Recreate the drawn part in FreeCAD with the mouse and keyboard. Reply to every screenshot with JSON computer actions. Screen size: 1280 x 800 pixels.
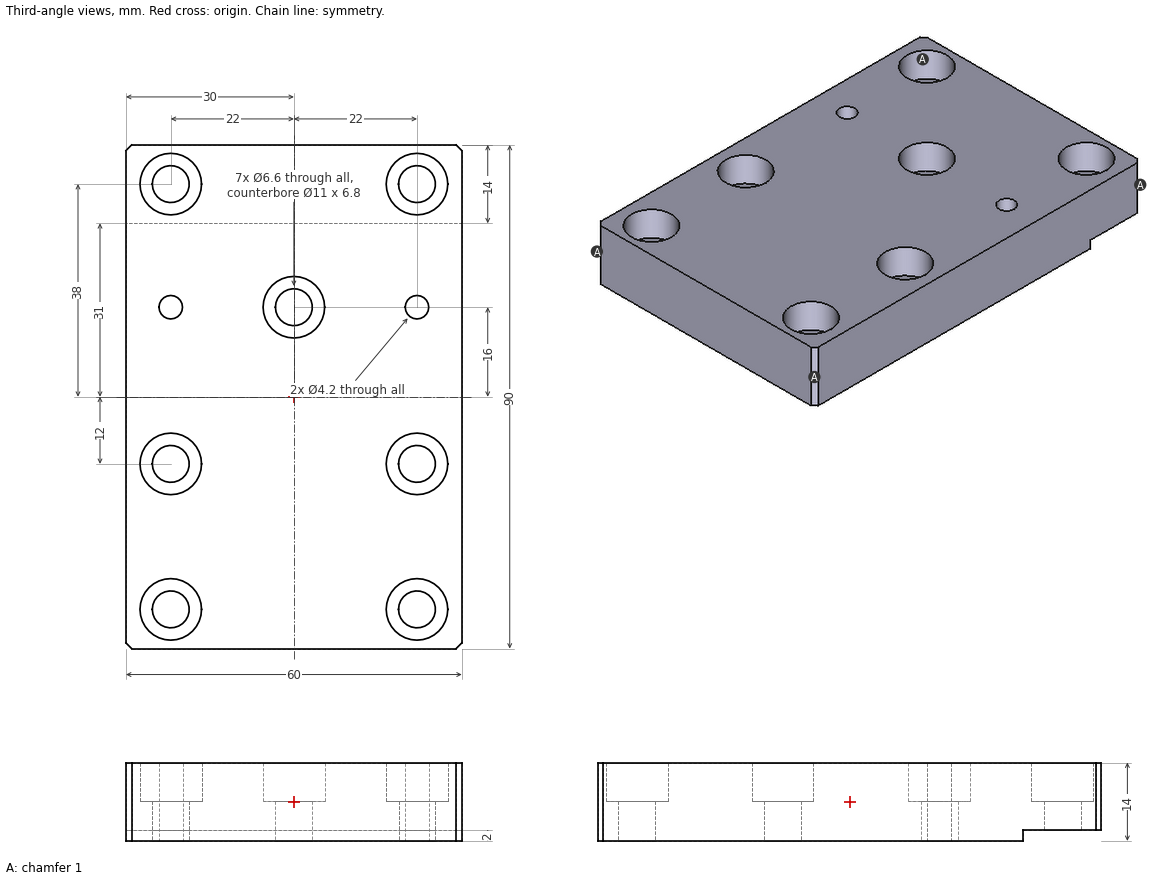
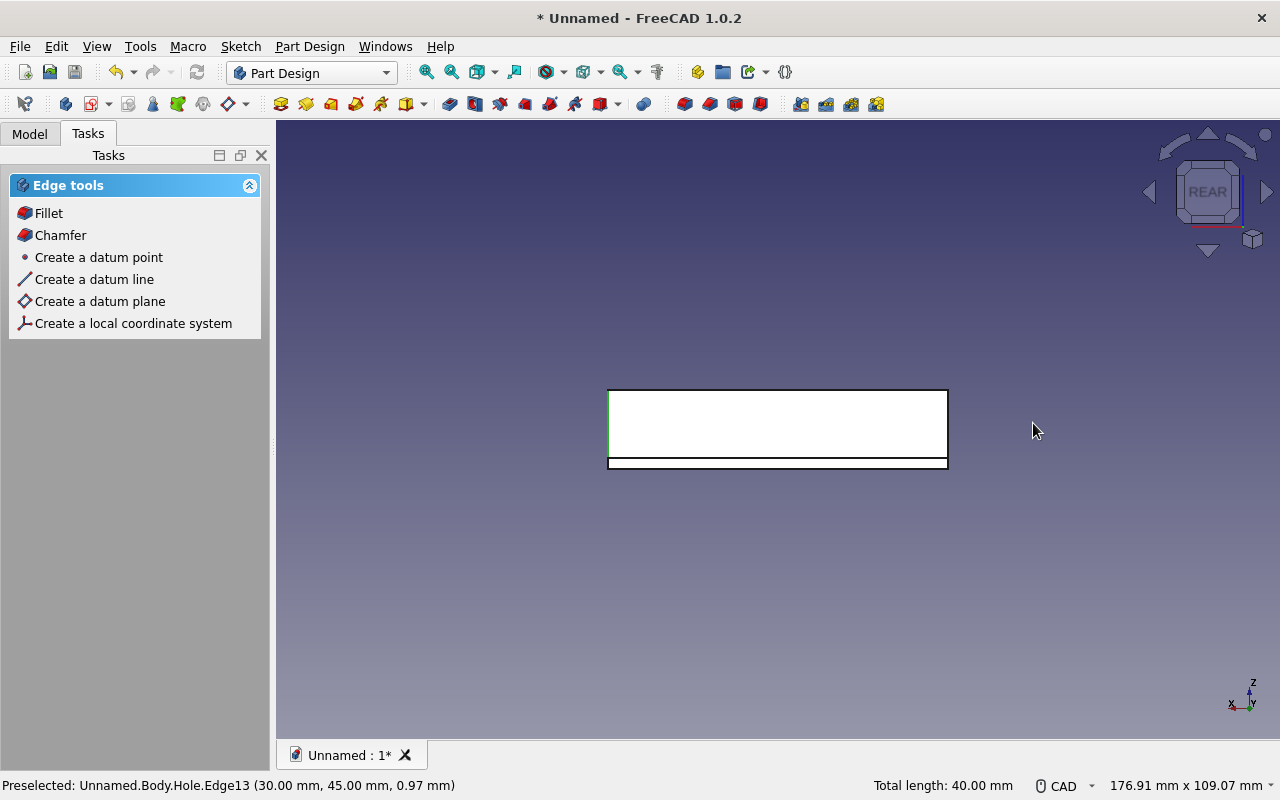
{"action": "left_click", "coordinate": [427, 72]}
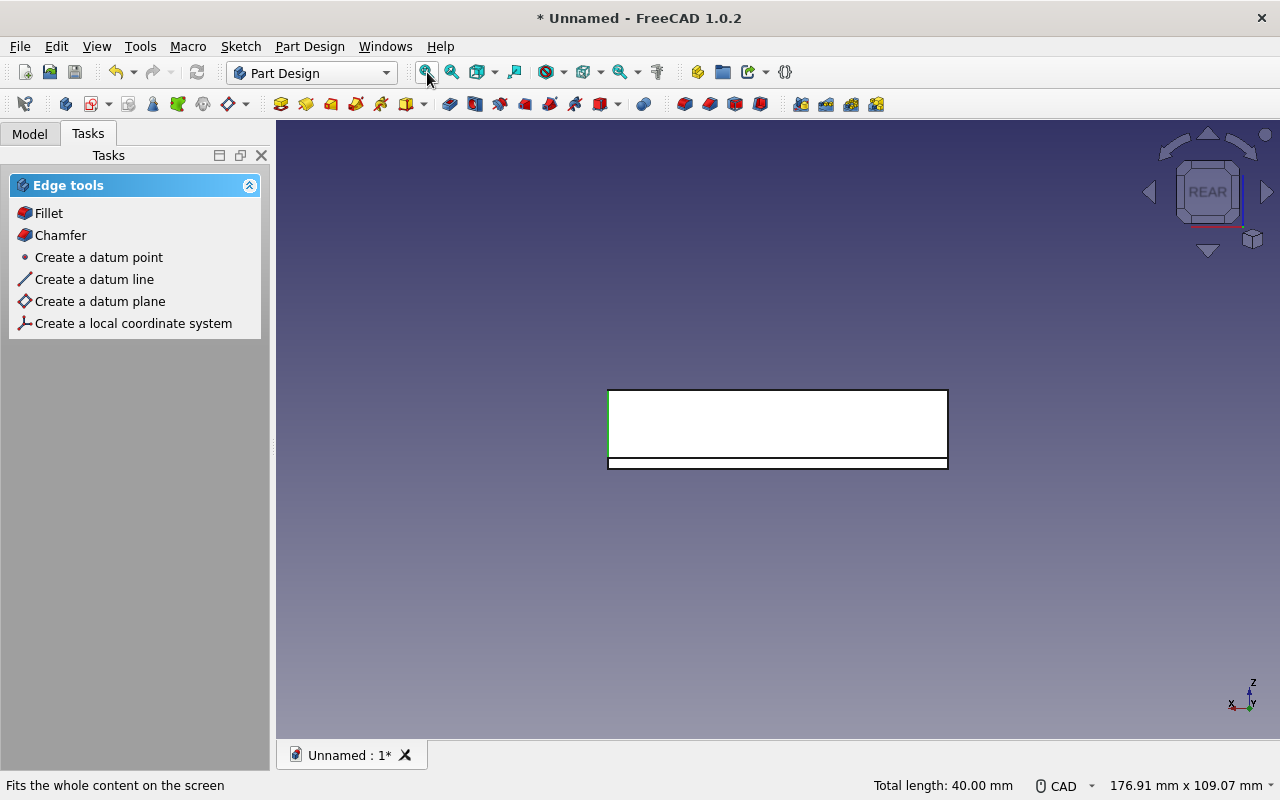
{"action": "left_click", "coordinate": [948, 423], "text": "ctrl"}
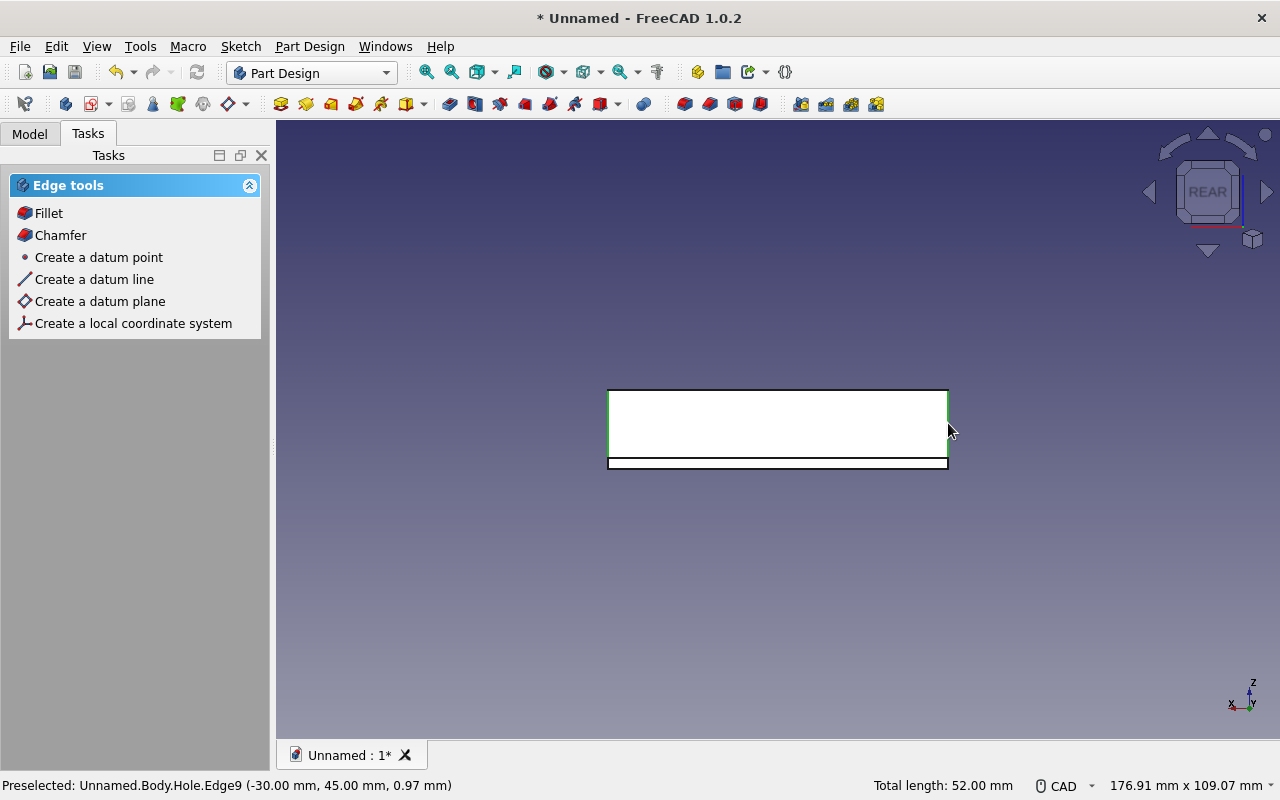
{"action": "left_click", "coordinate": [710, 104]}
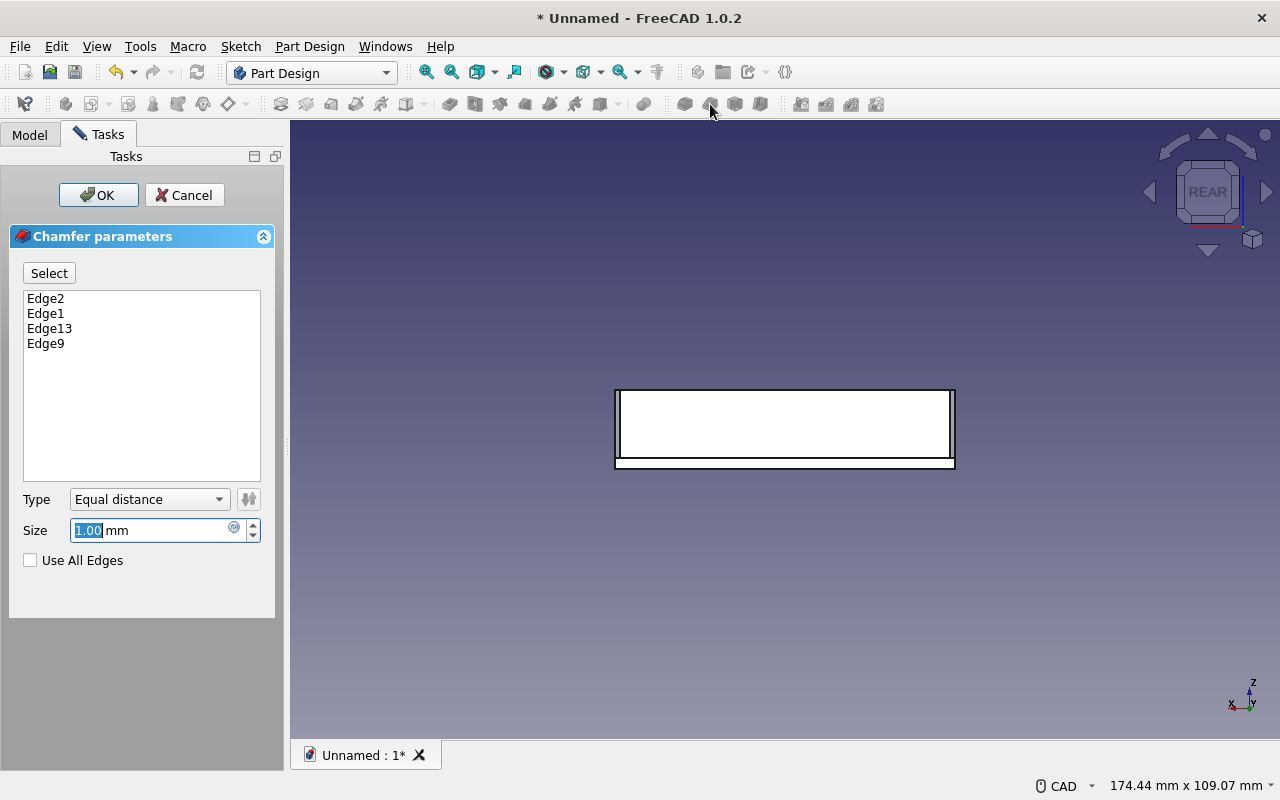
{"action": "type", "text": "1"}
{"action": "key", "text": "Tab"}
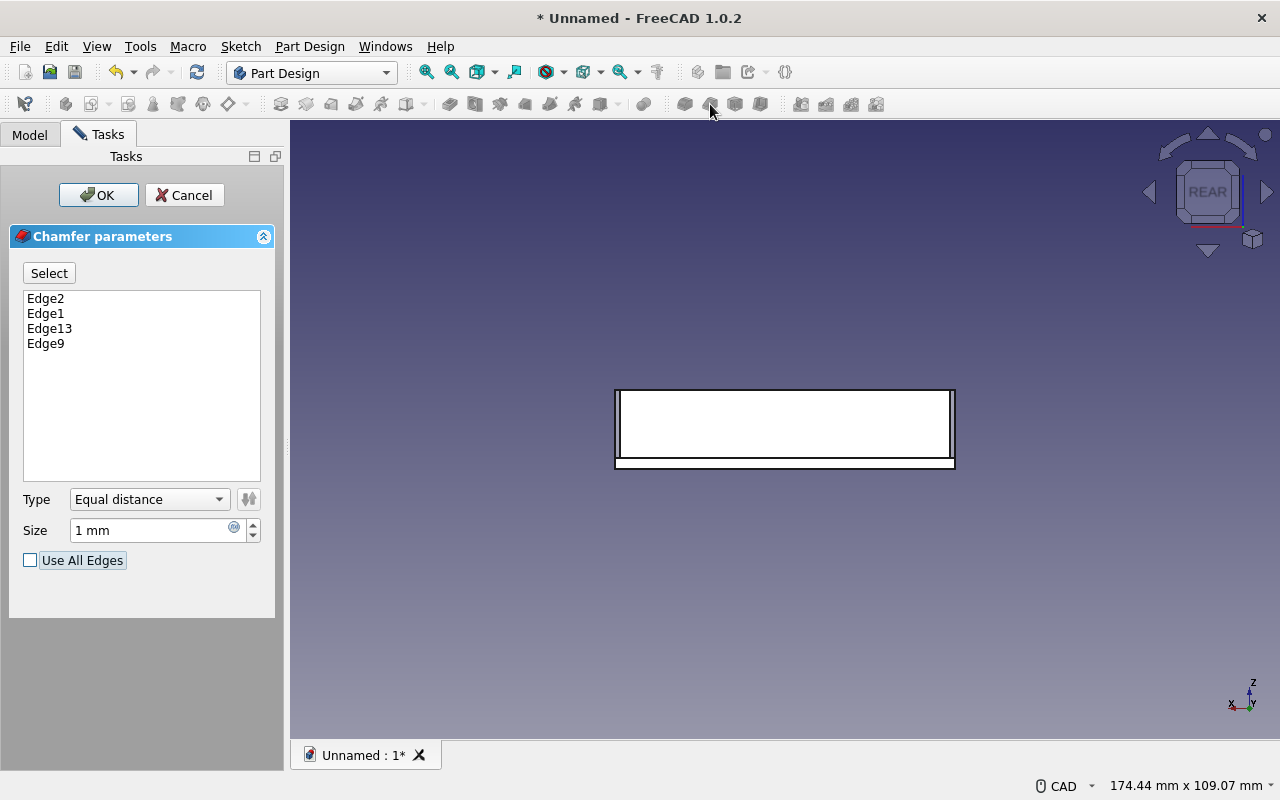
{"action": "left_click", "coordinate": [99, 195]}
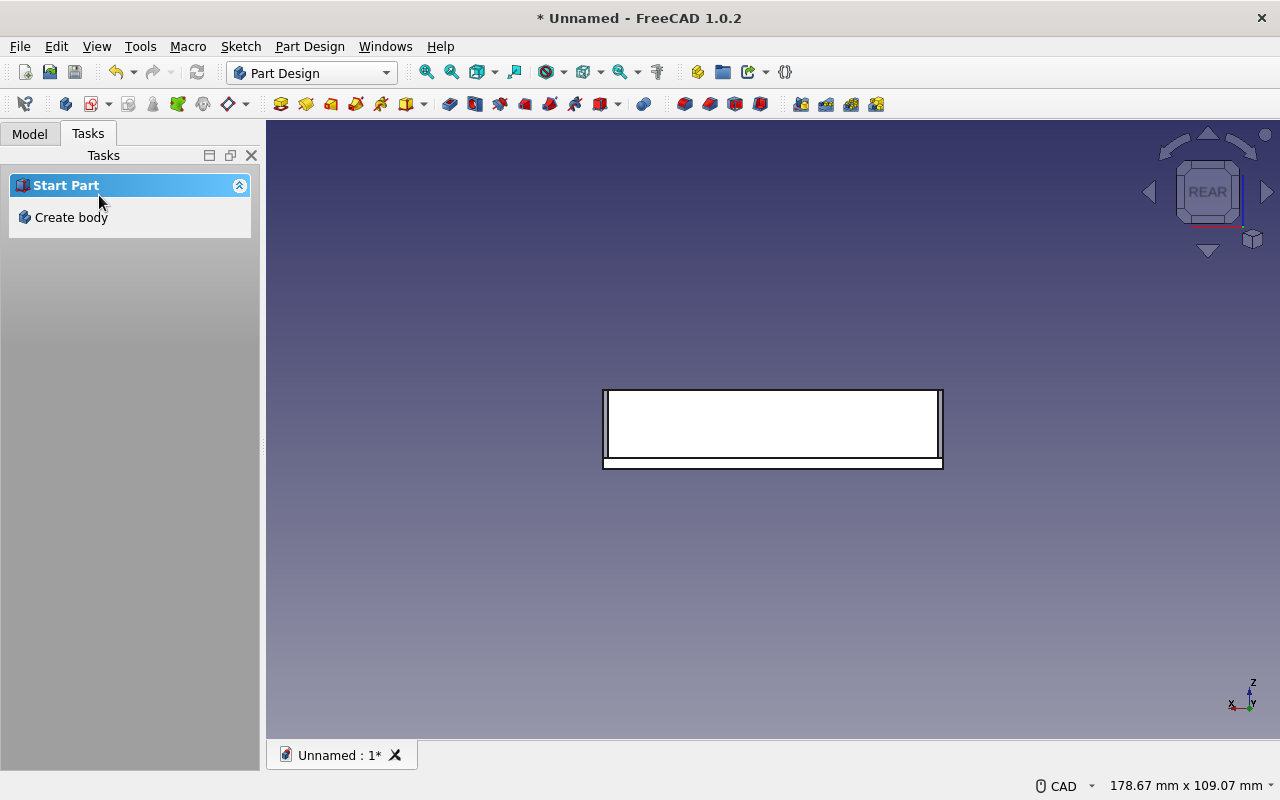
{"action": "left_click", "coordinate": [427, 72]}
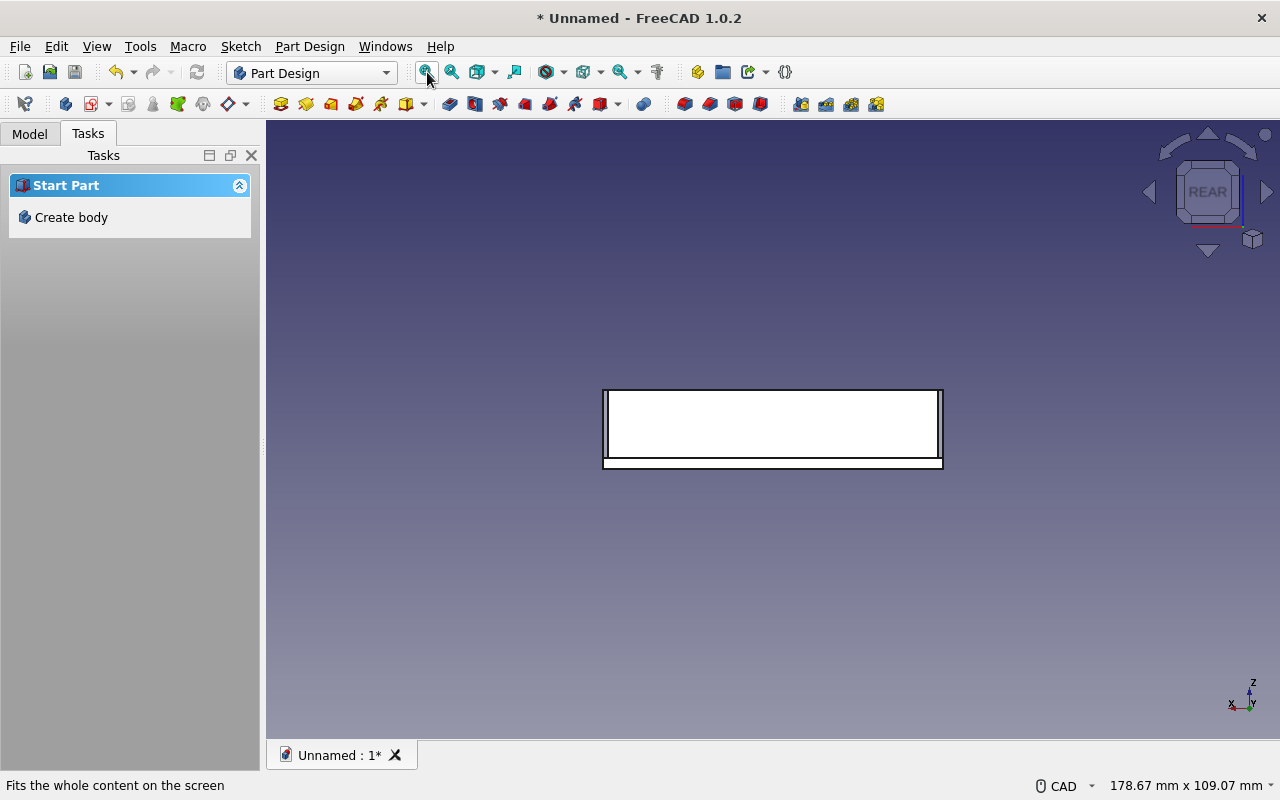
{"action": "key", "text": "0"}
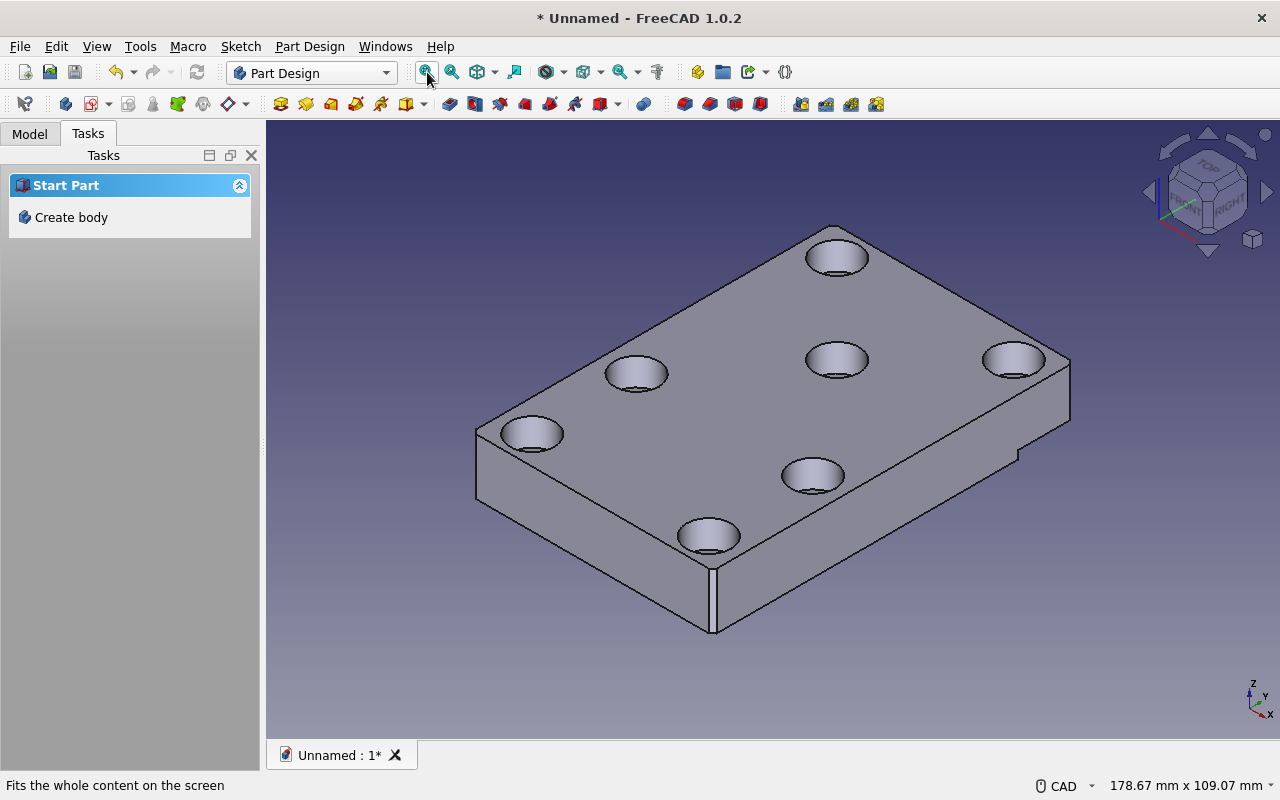
{"action": "left_click", "coordinate": [670, 456]}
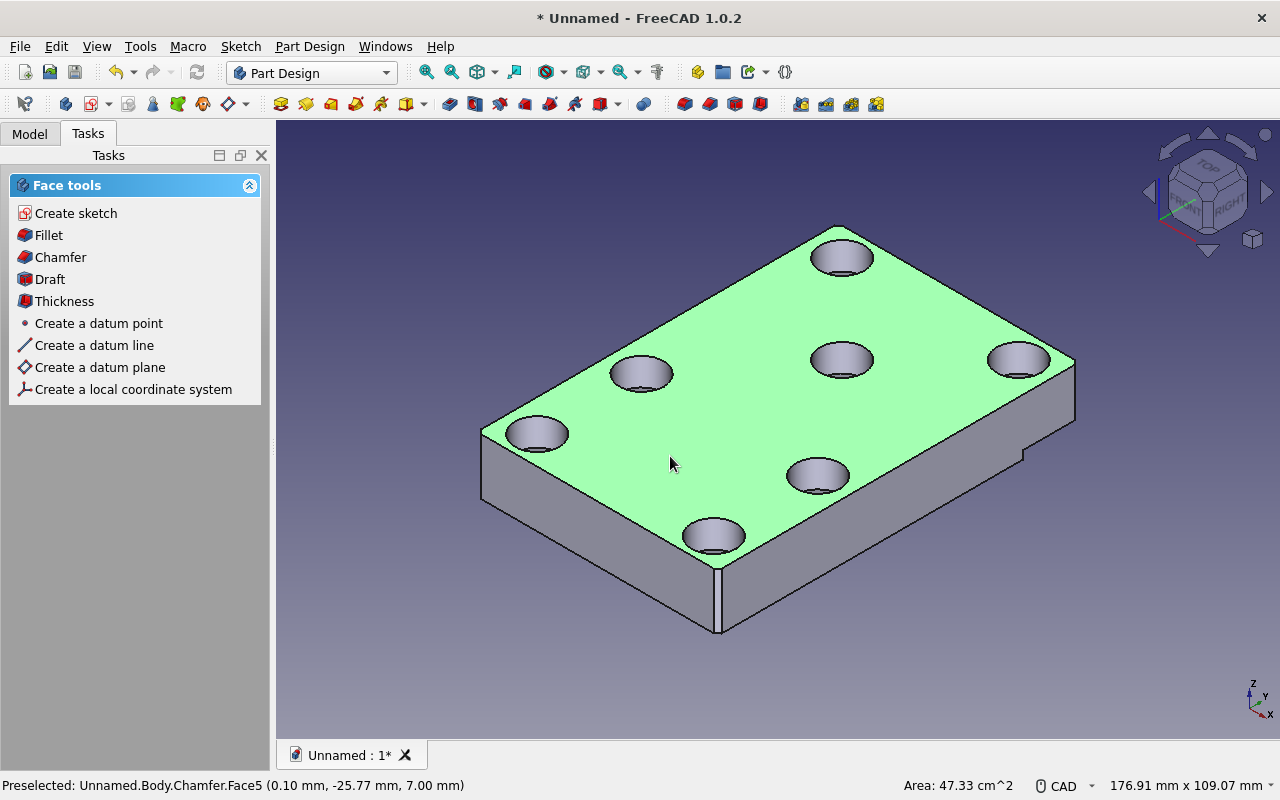
{"action": "left_click", "coordinate": [90, 104]}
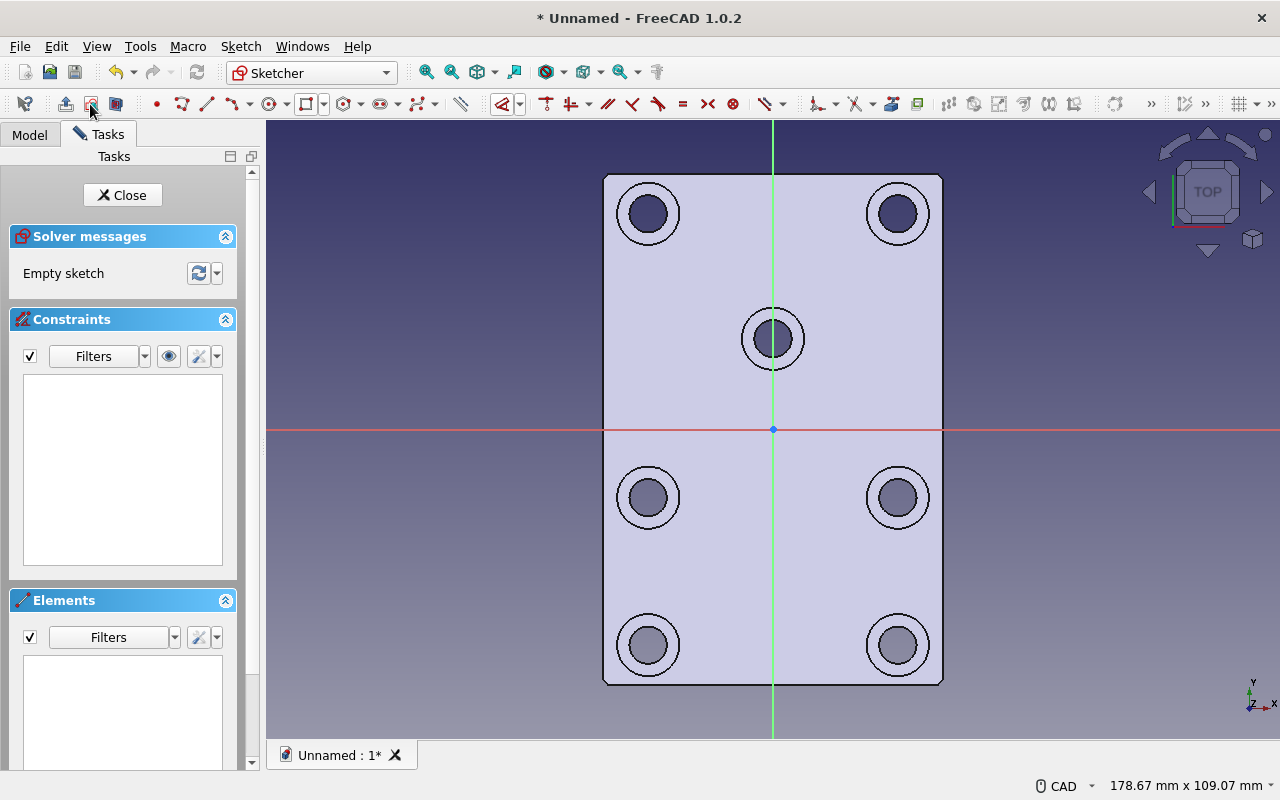
{"action": "scroll", "coordinate": [829, 336], "scroll_direction": "up", "scroll_amount": 4}